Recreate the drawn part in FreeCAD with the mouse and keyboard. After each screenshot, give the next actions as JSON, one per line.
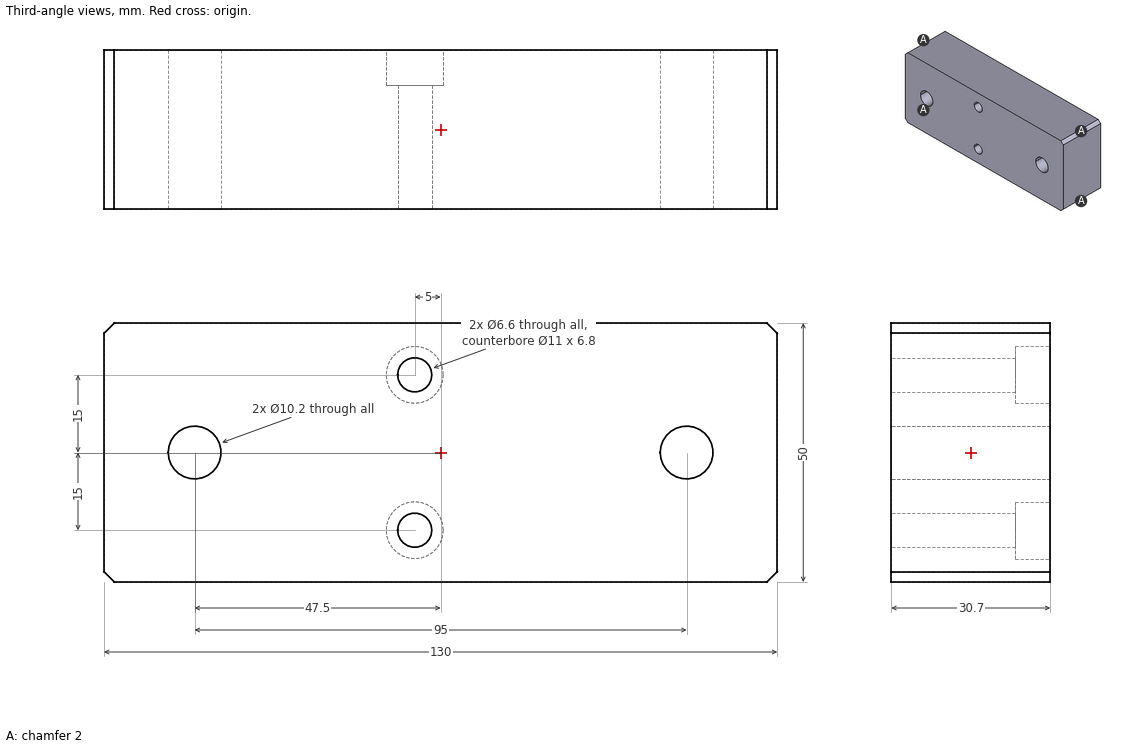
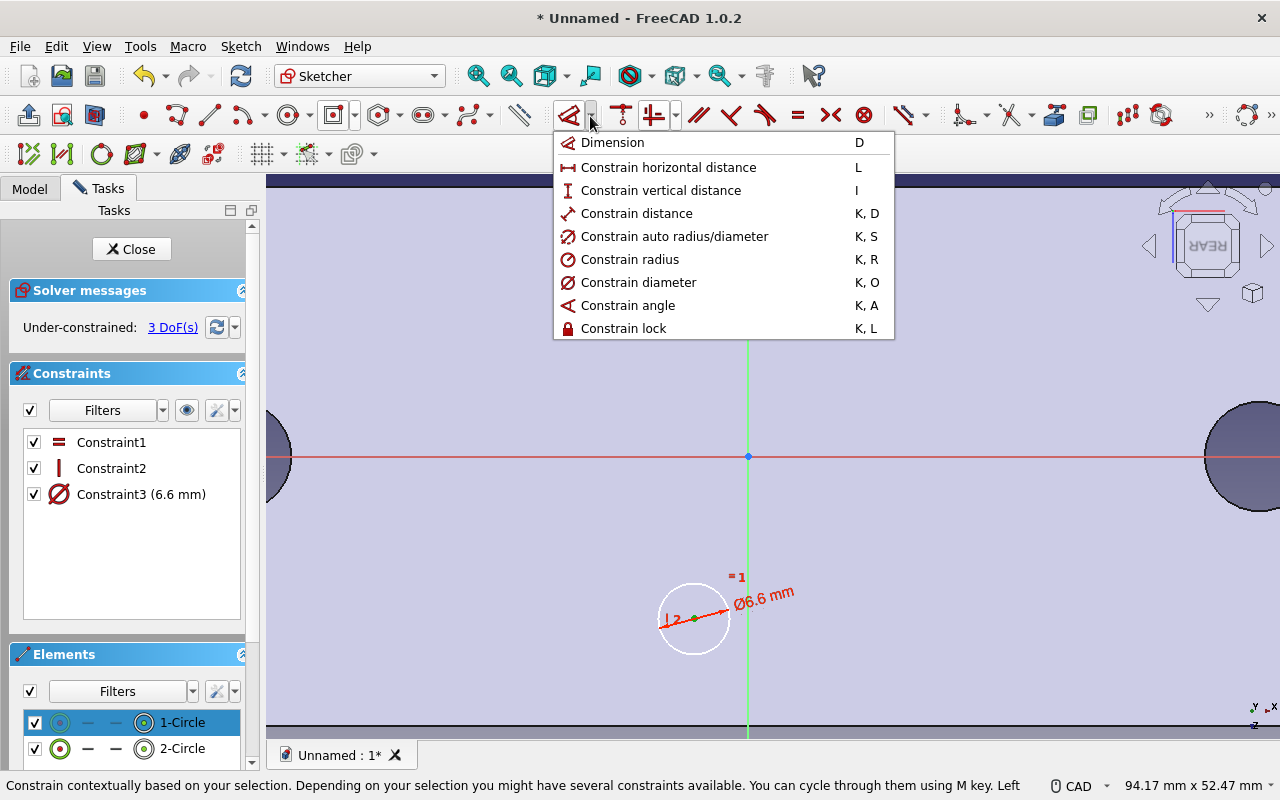
{"action": "left_click", "coordinate": [724, 168]}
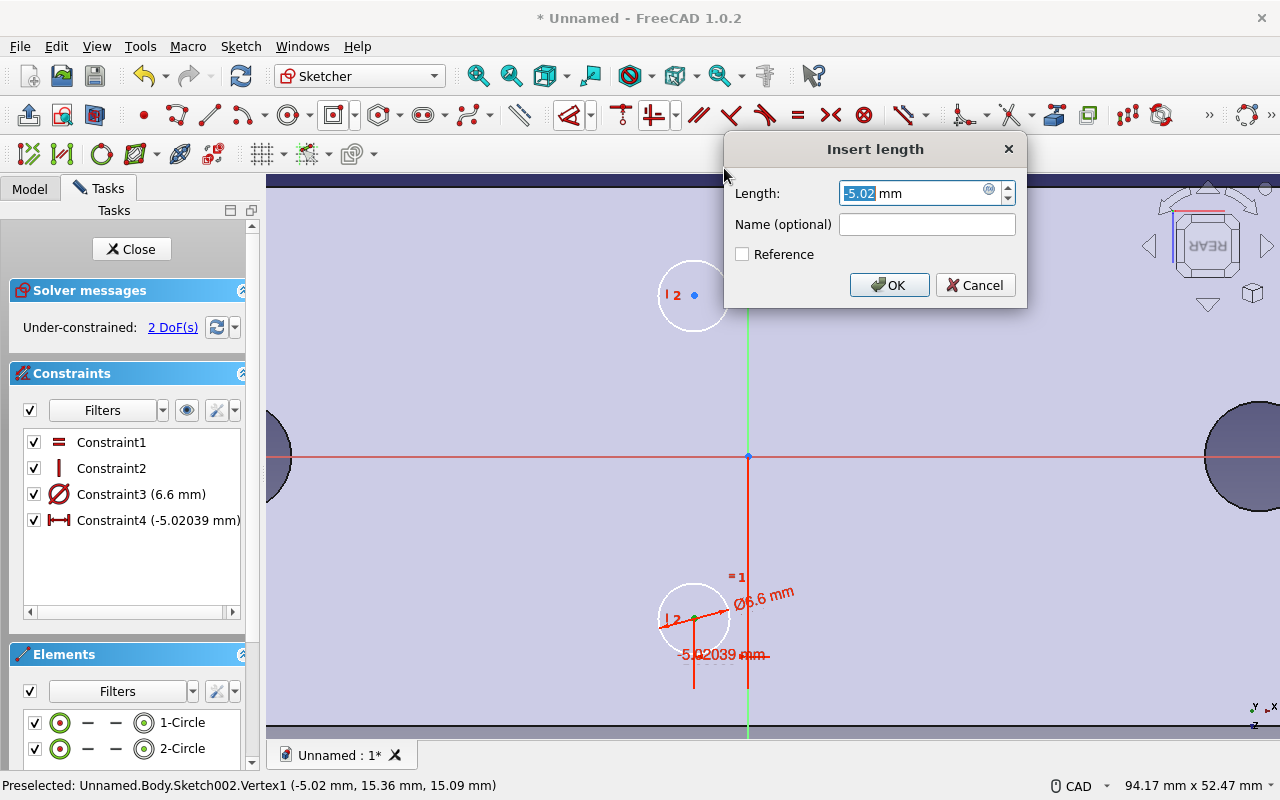
{"action": "type", "text": "-5"}
{"action": "key", "text": "Return"}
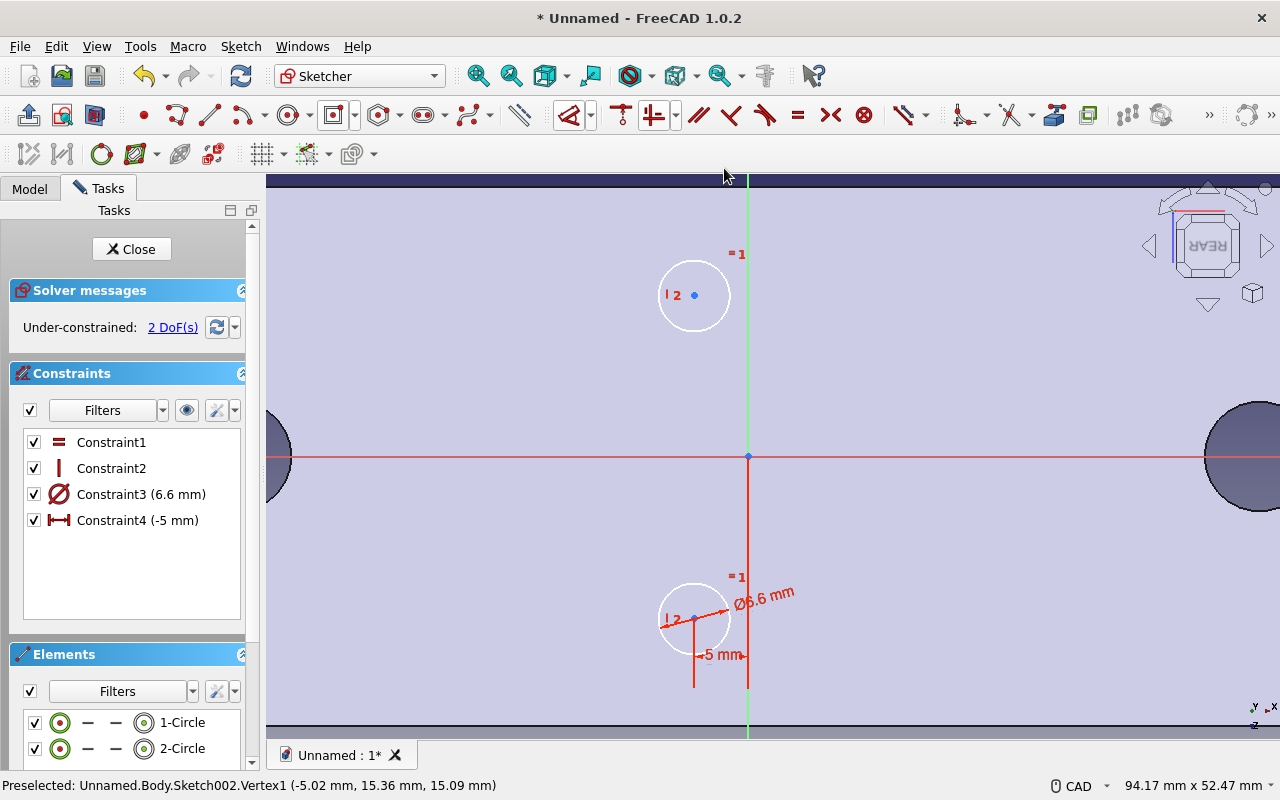
{"action": "left_click", "coordinate": [694, 619]}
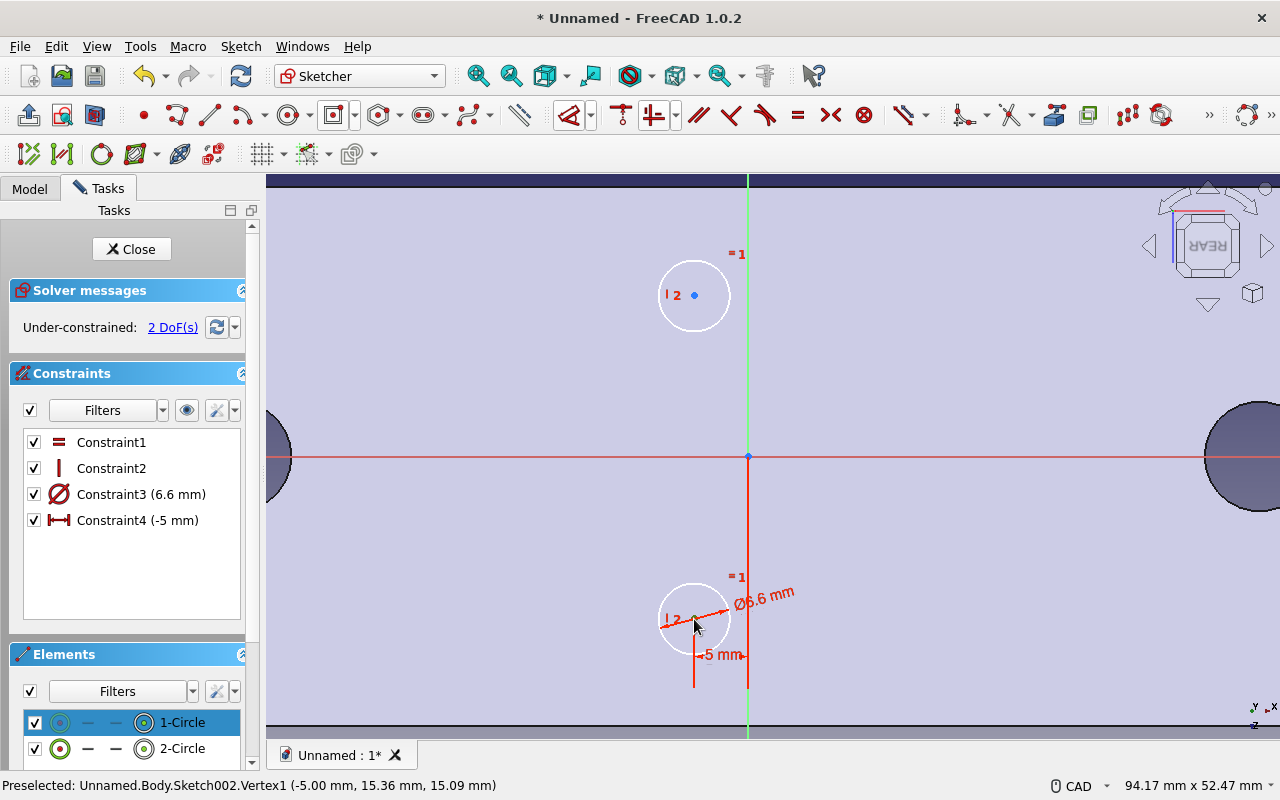
{"action": "key", "text": "i"}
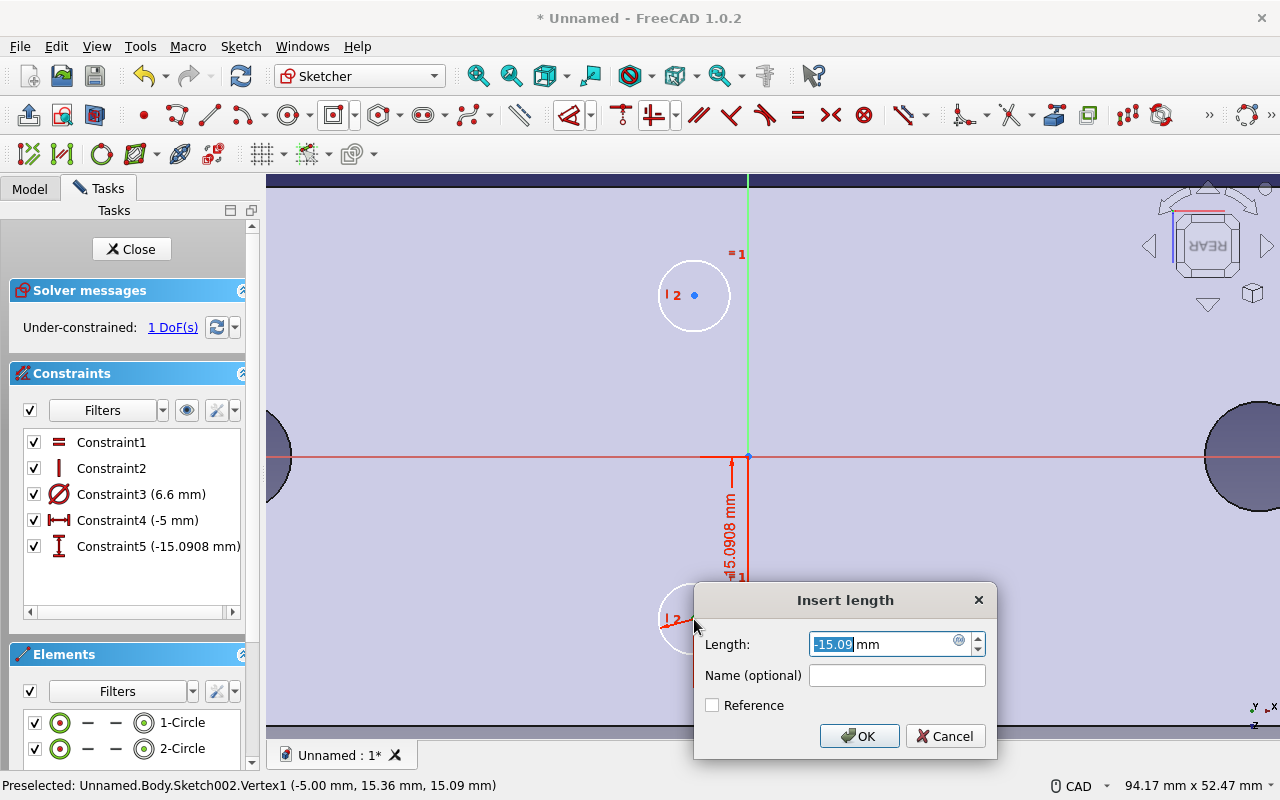
{"action": "type", "text": "-15"}
{"action": "key", "text": "Return"}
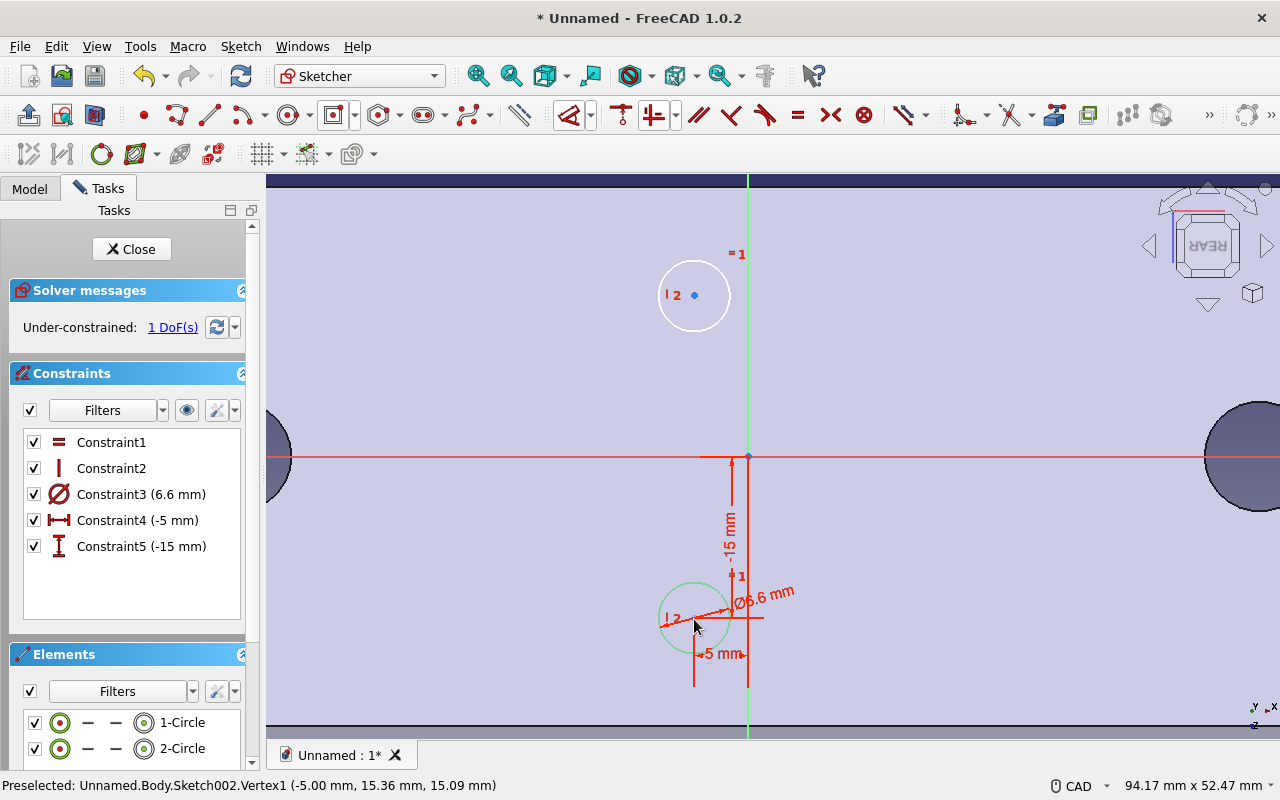
{"action": "left_click", "coordinate": [694, 296]}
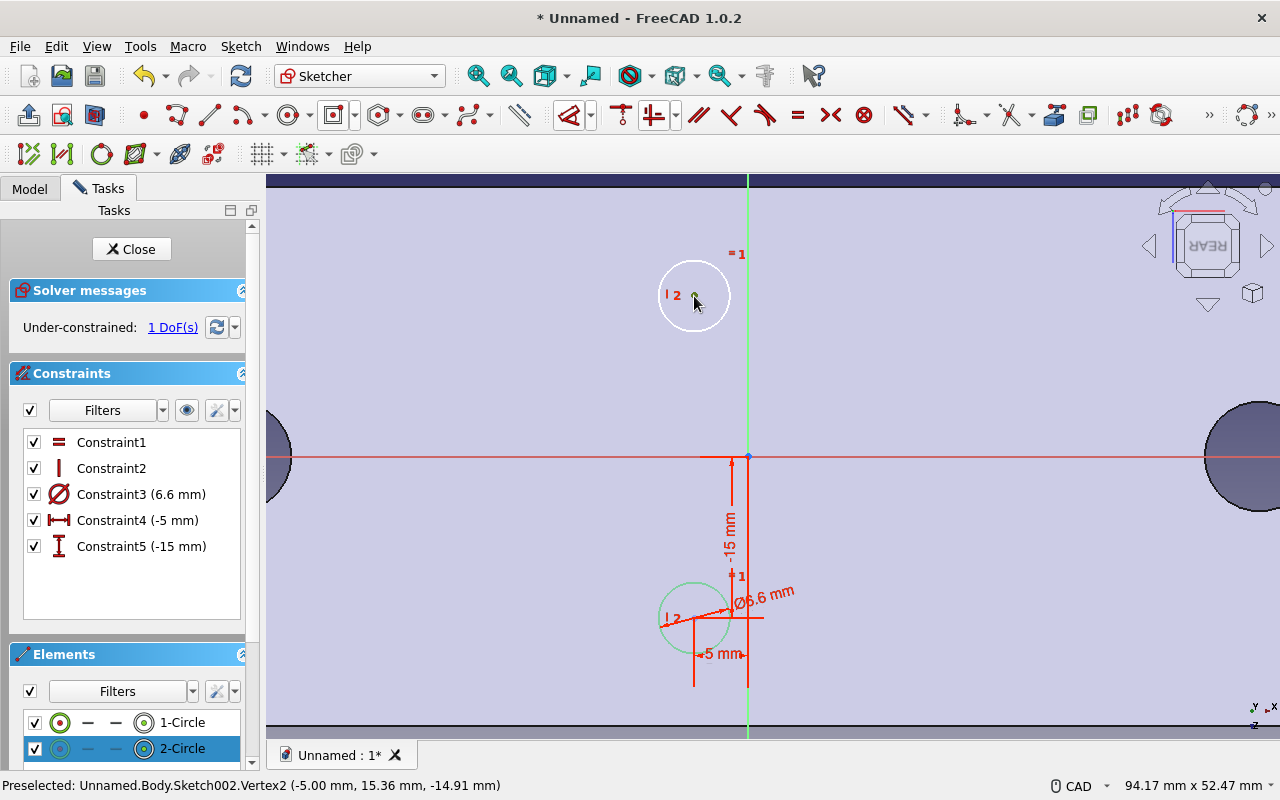
{"action": "key", "text": "i"}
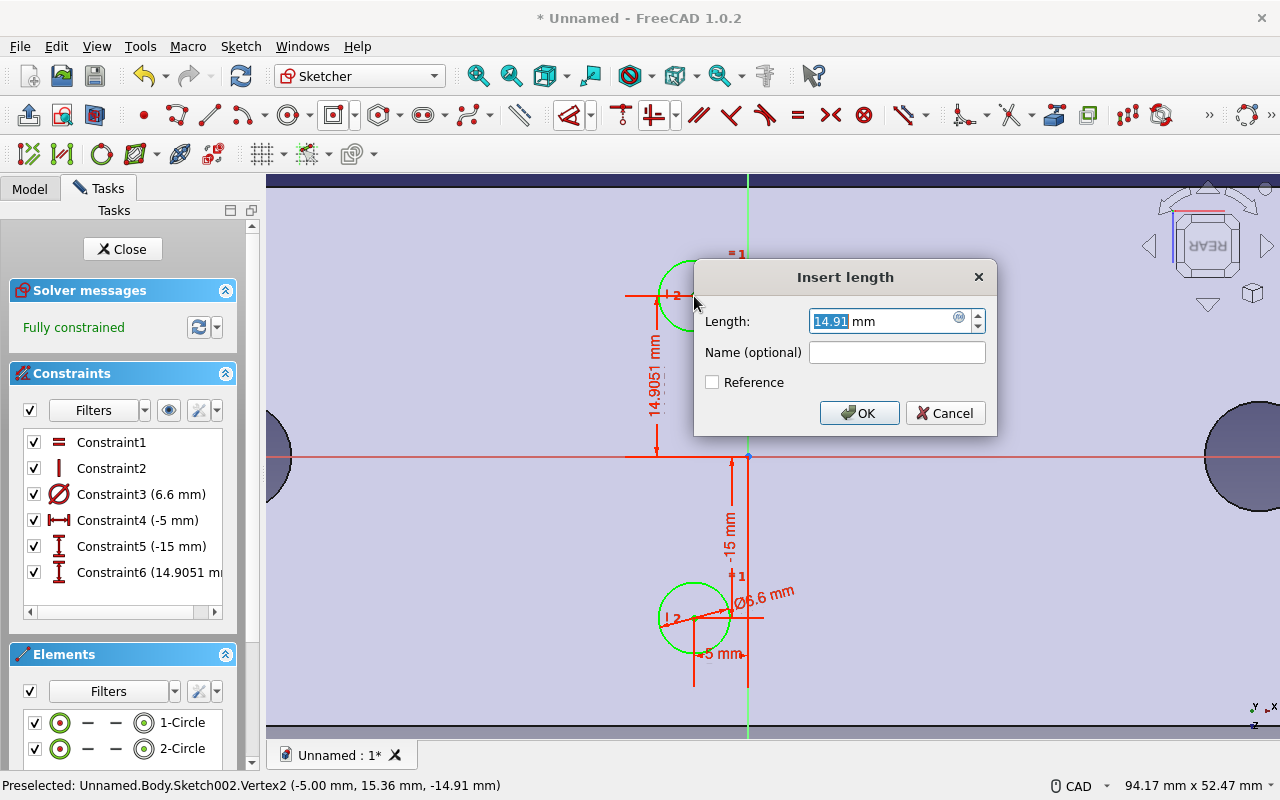
{"action": "type", "text": "15"}
{"action": "key", "text": "Return"}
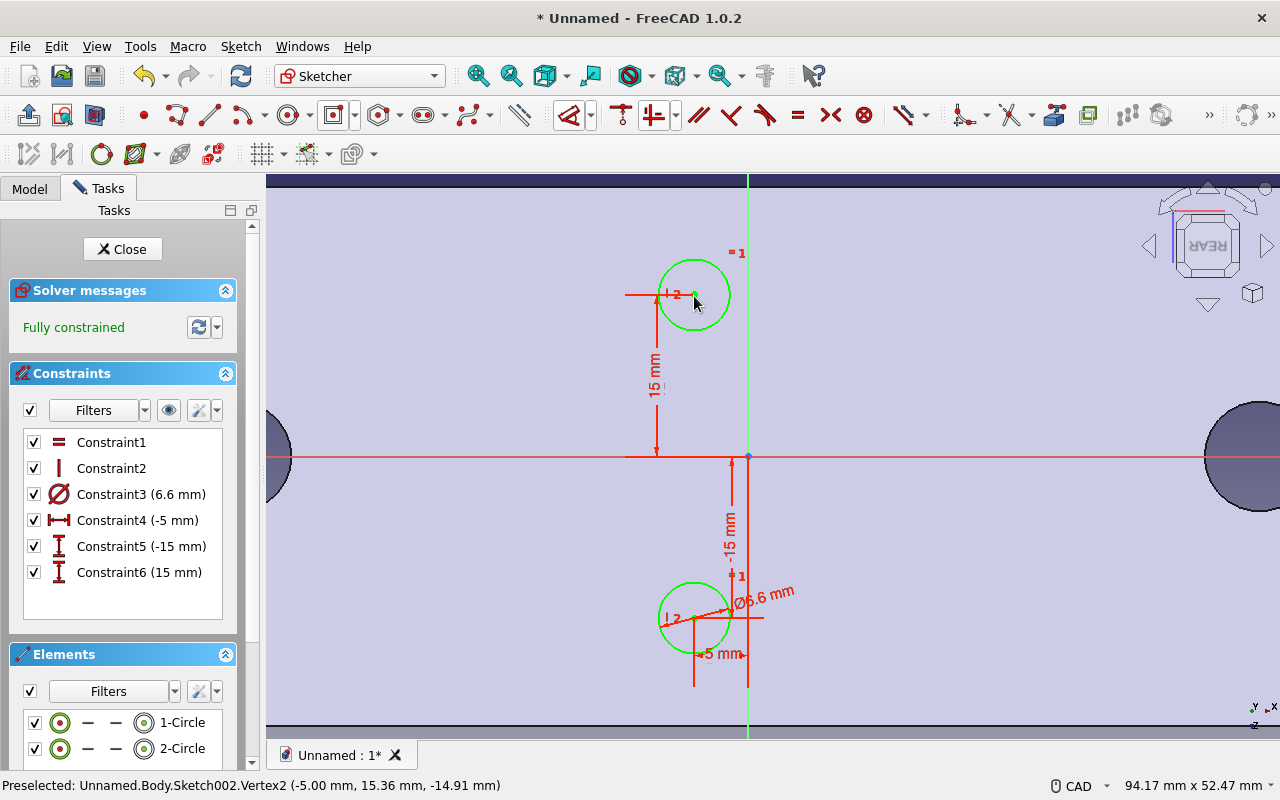
{"action": "left_click", "coordinate": [123, 249]}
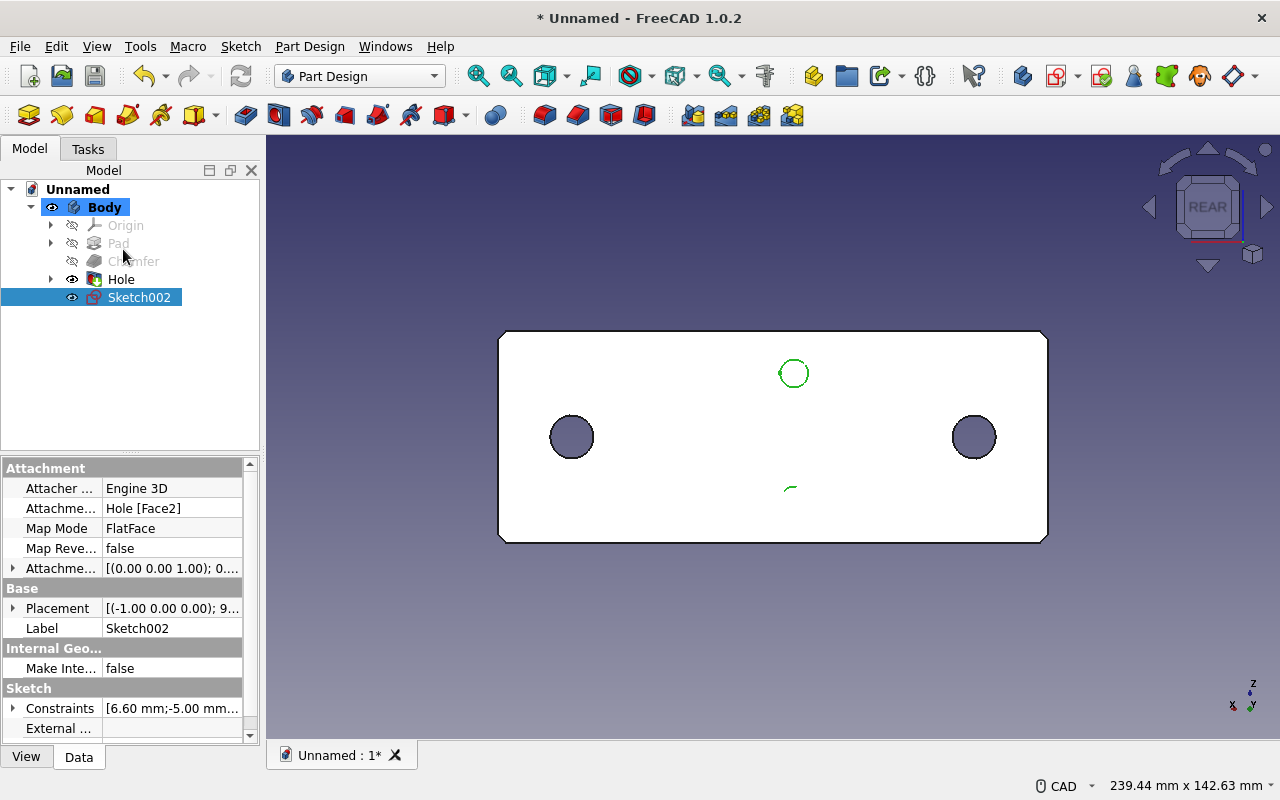
{"action": "left_click", "coordinate": [279, 116]}